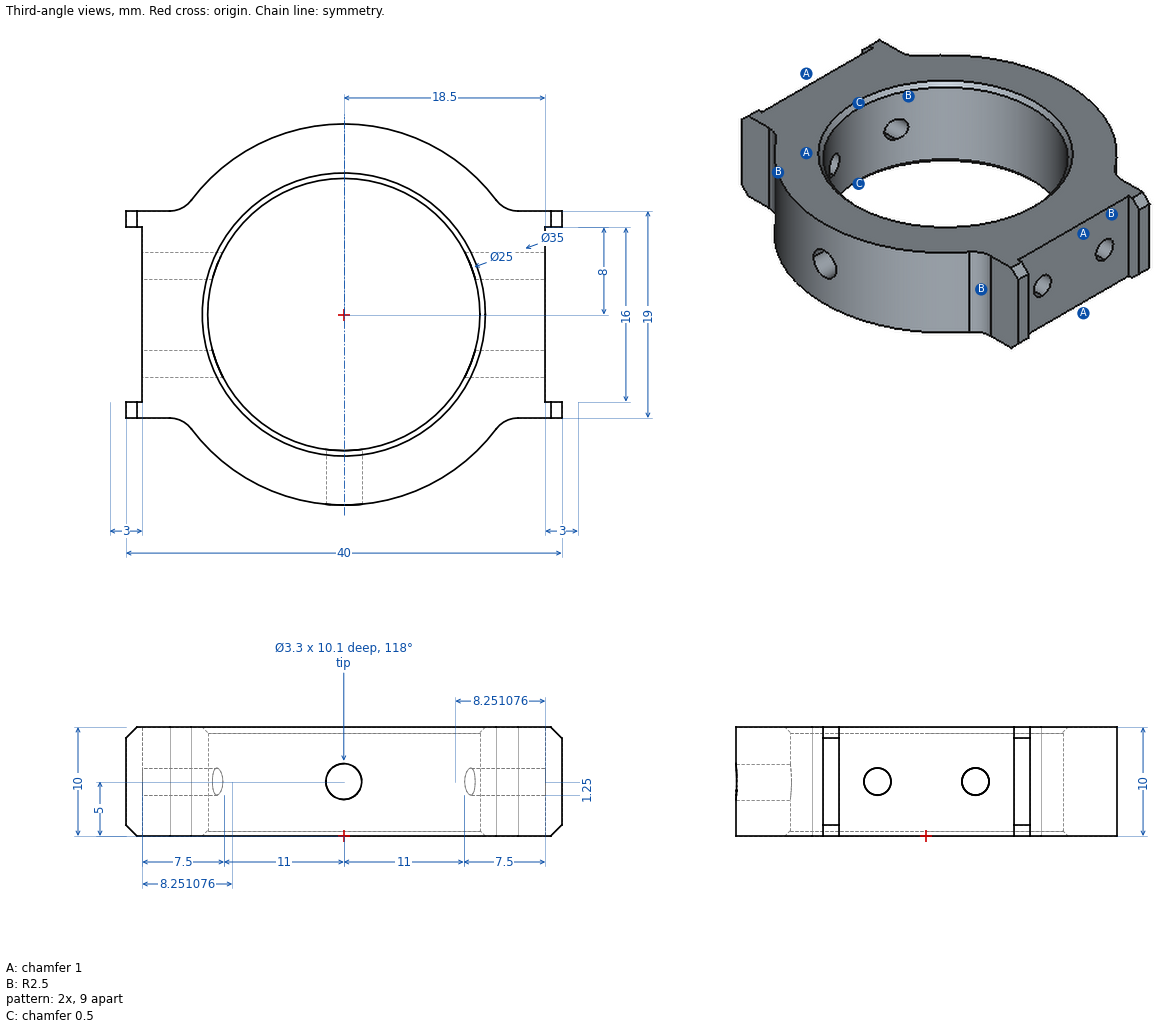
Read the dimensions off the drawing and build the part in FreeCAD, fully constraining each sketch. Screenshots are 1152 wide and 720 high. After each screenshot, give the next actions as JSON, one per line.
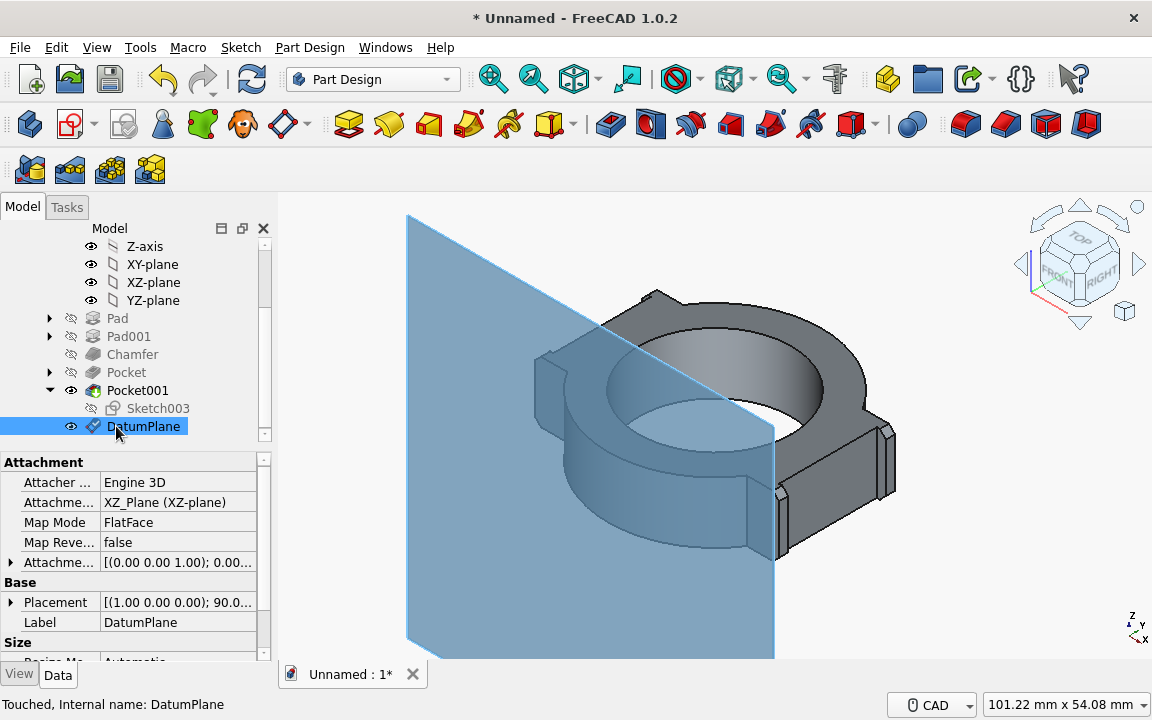
{"action": "left_click", "coordinate": [70, 124]}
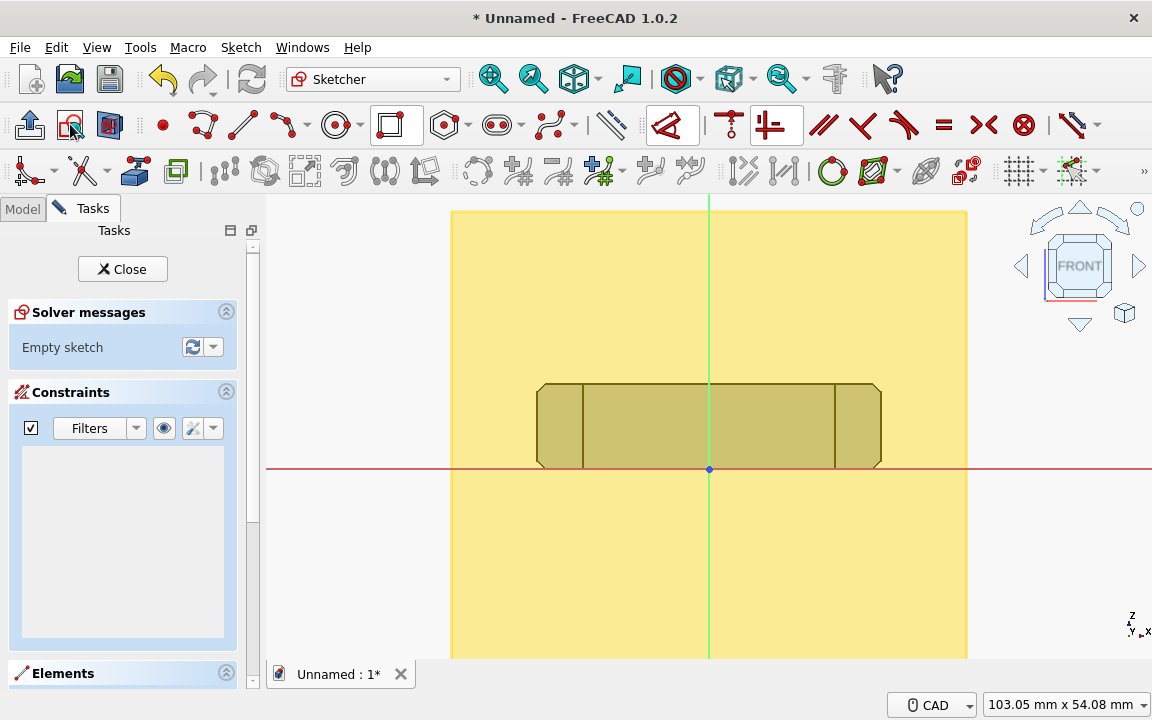
{"action": "scroll", "coordinate": [726, 445], "scroll_direction": "up", "scroll_amount": 8}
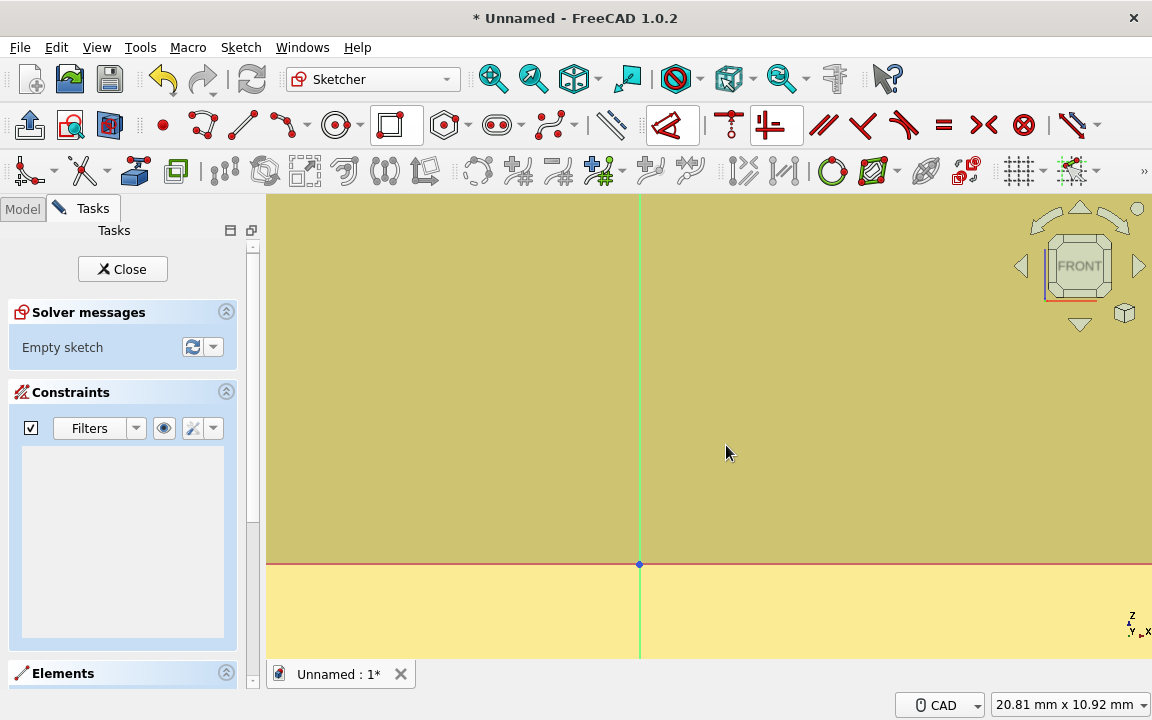
{"action": "key", "text": "g c"}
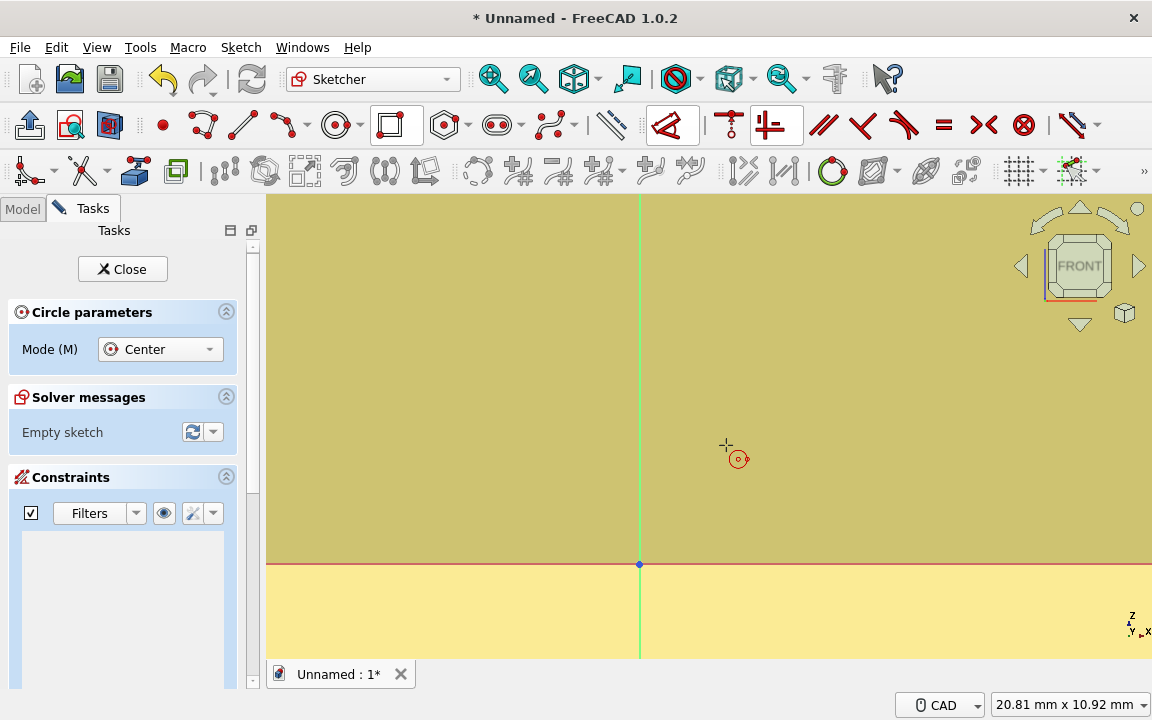
{"action": "left_click", "coordinate": [640, 351]}
{"action": "mouse_move", "coordinate": [689, 302]}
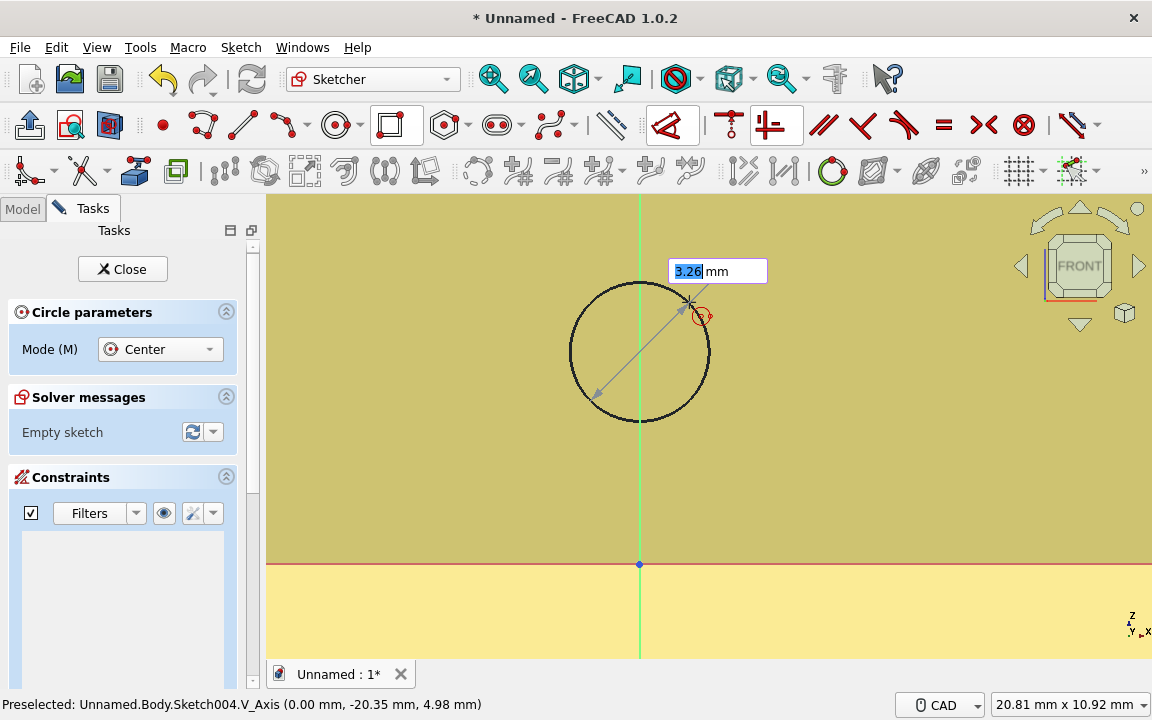
{"action": "type", "text": "3.3"}
{"action": "key", "text": "Return"}
{"action": "key", "text": "Escape"}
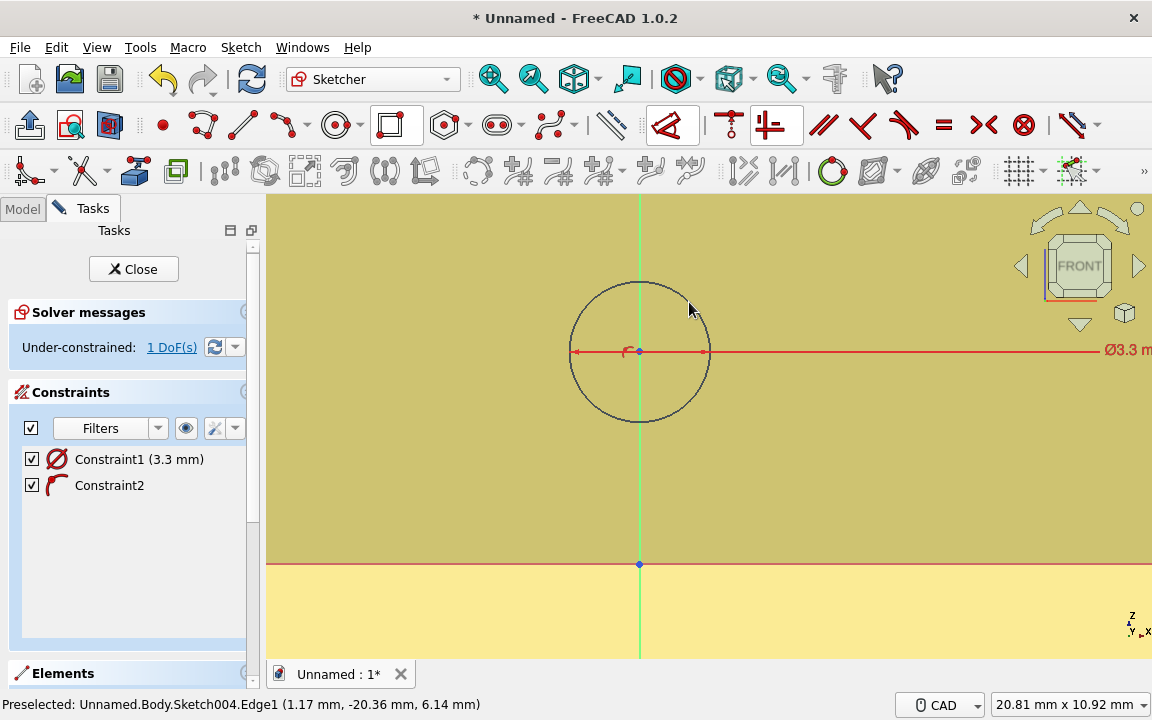
{"action": "left_click", "coordinate": [640, 352]}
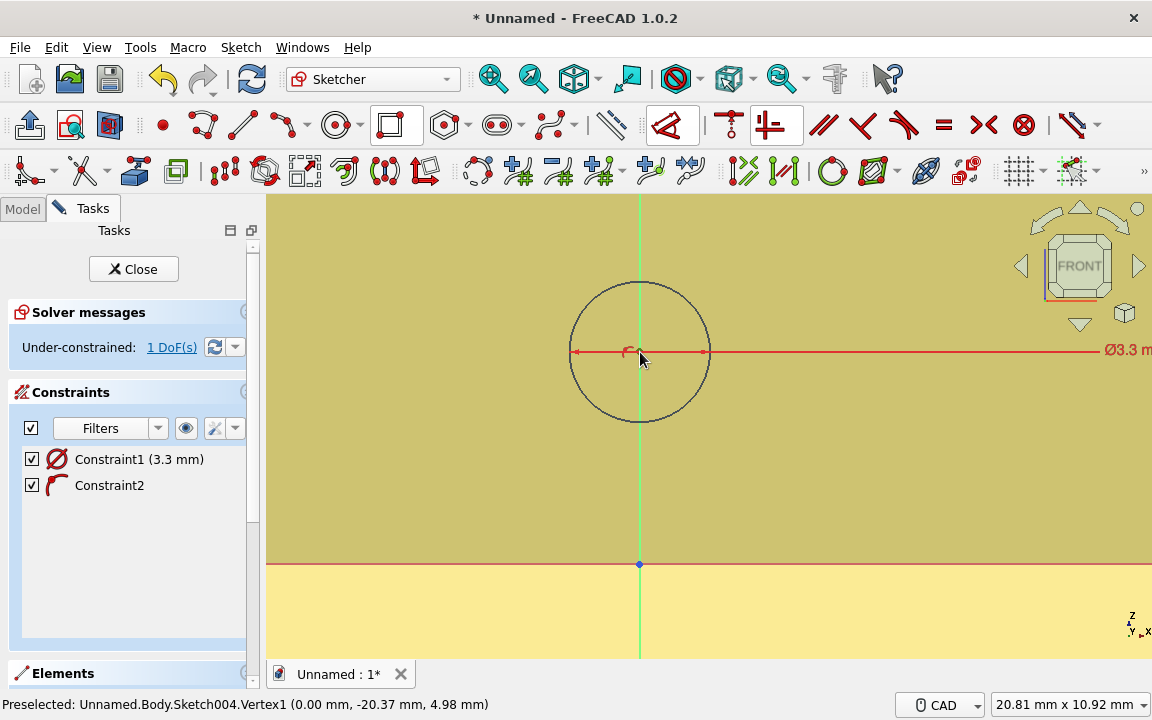
{"action": "key", "text": "i"}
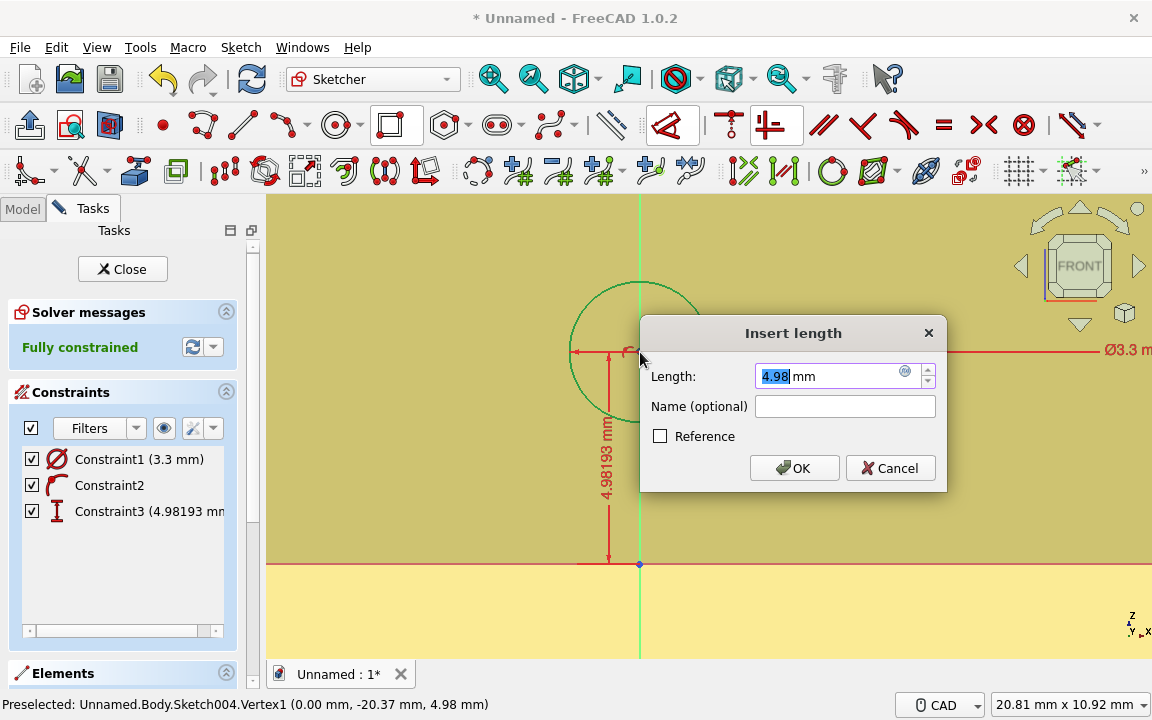
{"action": "type", "text": "5"}
{"action": "key", "text": "Return"}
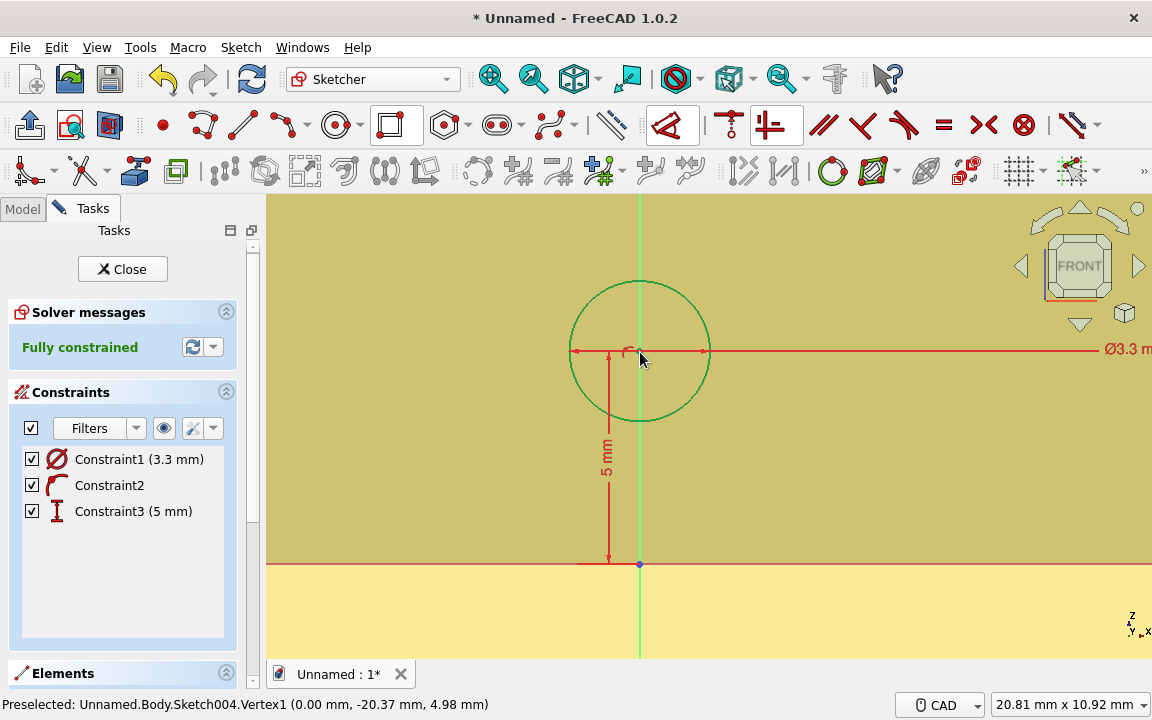
{"action": "left_click", "coordinate": [123, 269]}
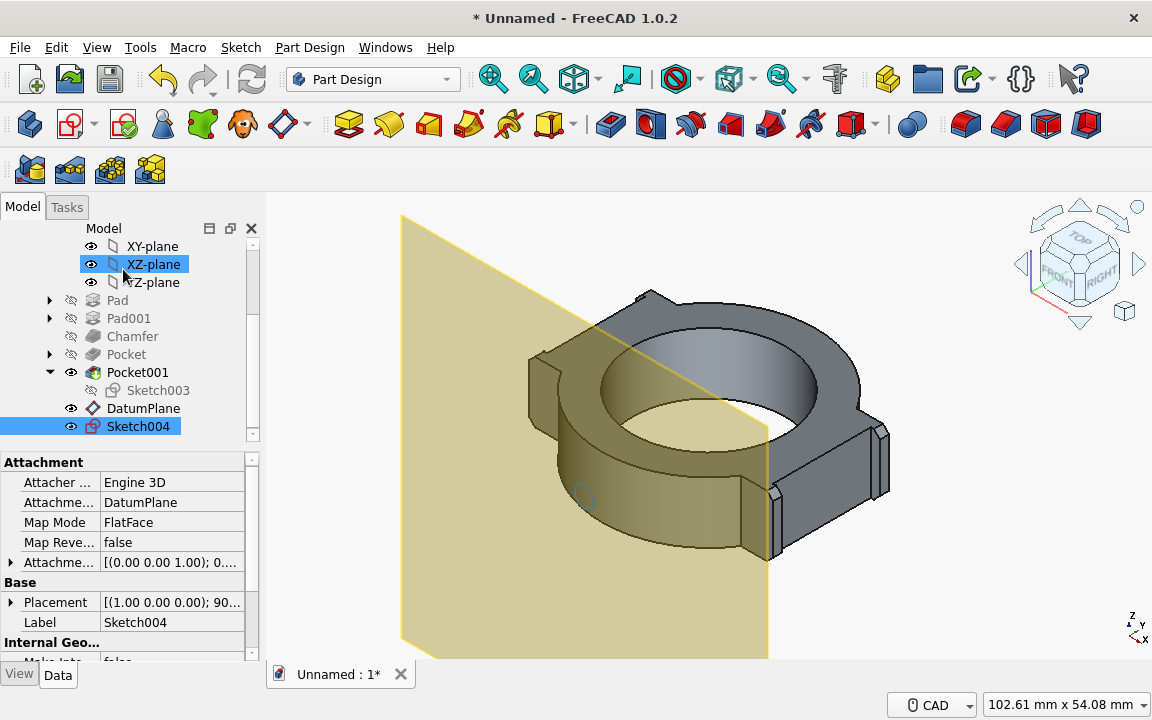
{"action": "left_click", "coordinate": [652, 124]}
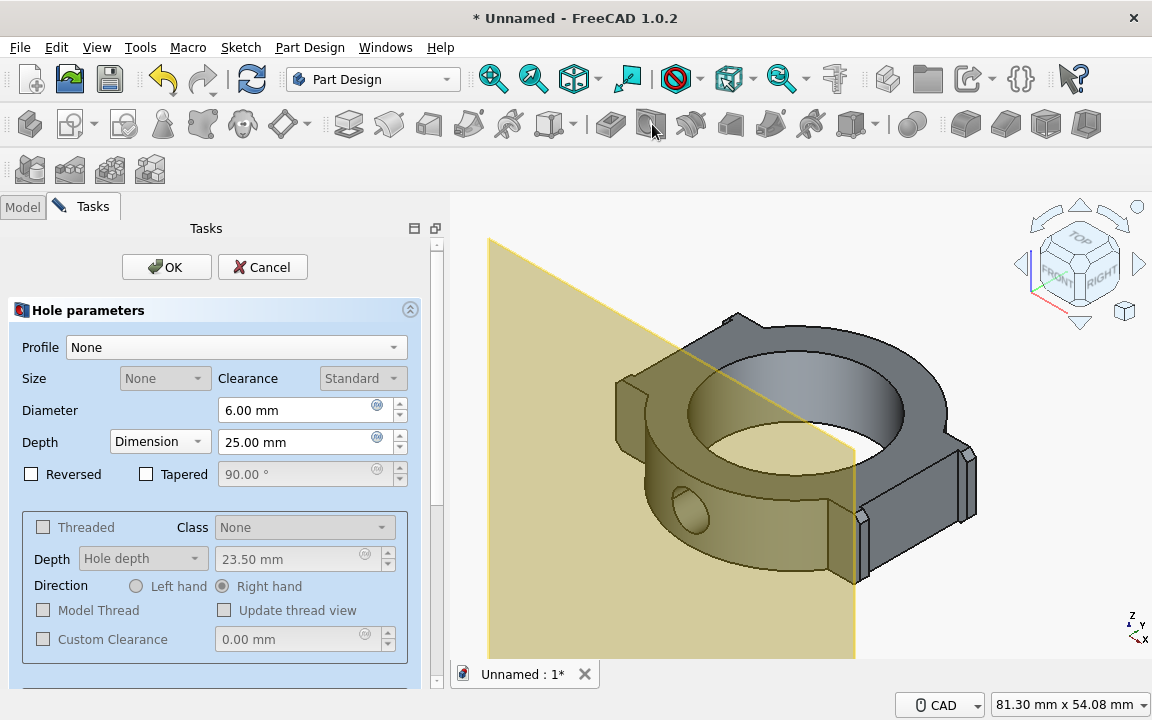
{"action": "triple_click", "coordinate": [305, 410]}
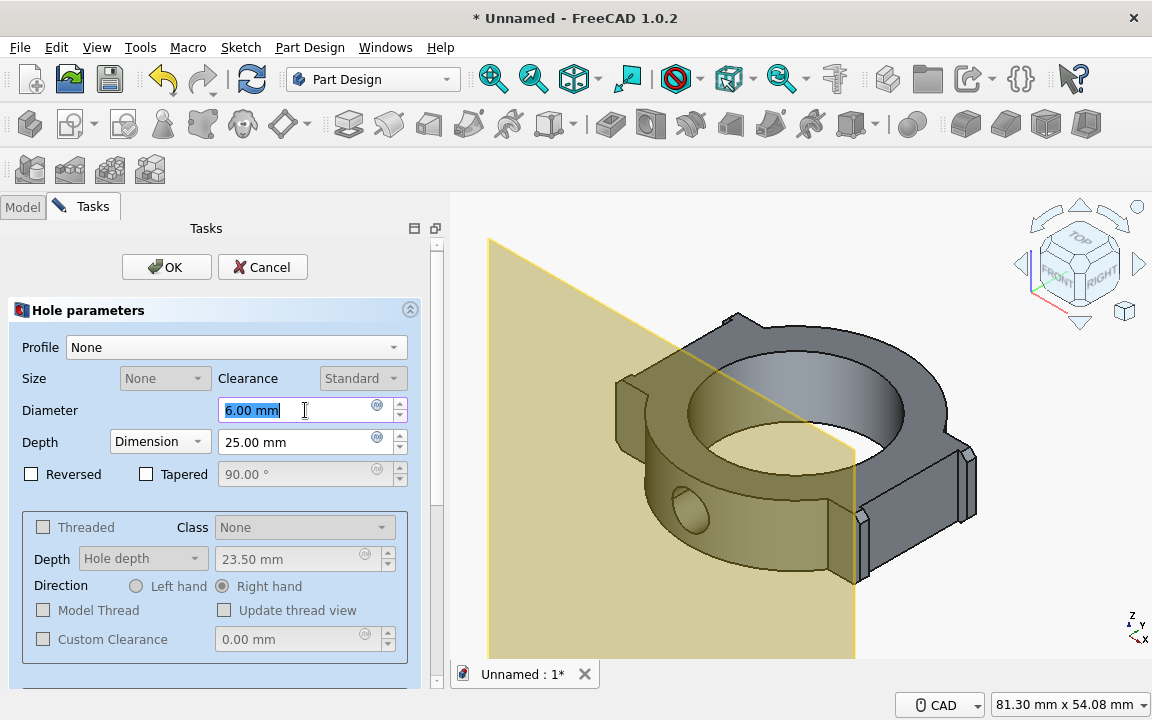
{"action": "type", "text": "3.3"}
{"action": "key", "text": "Tab"}